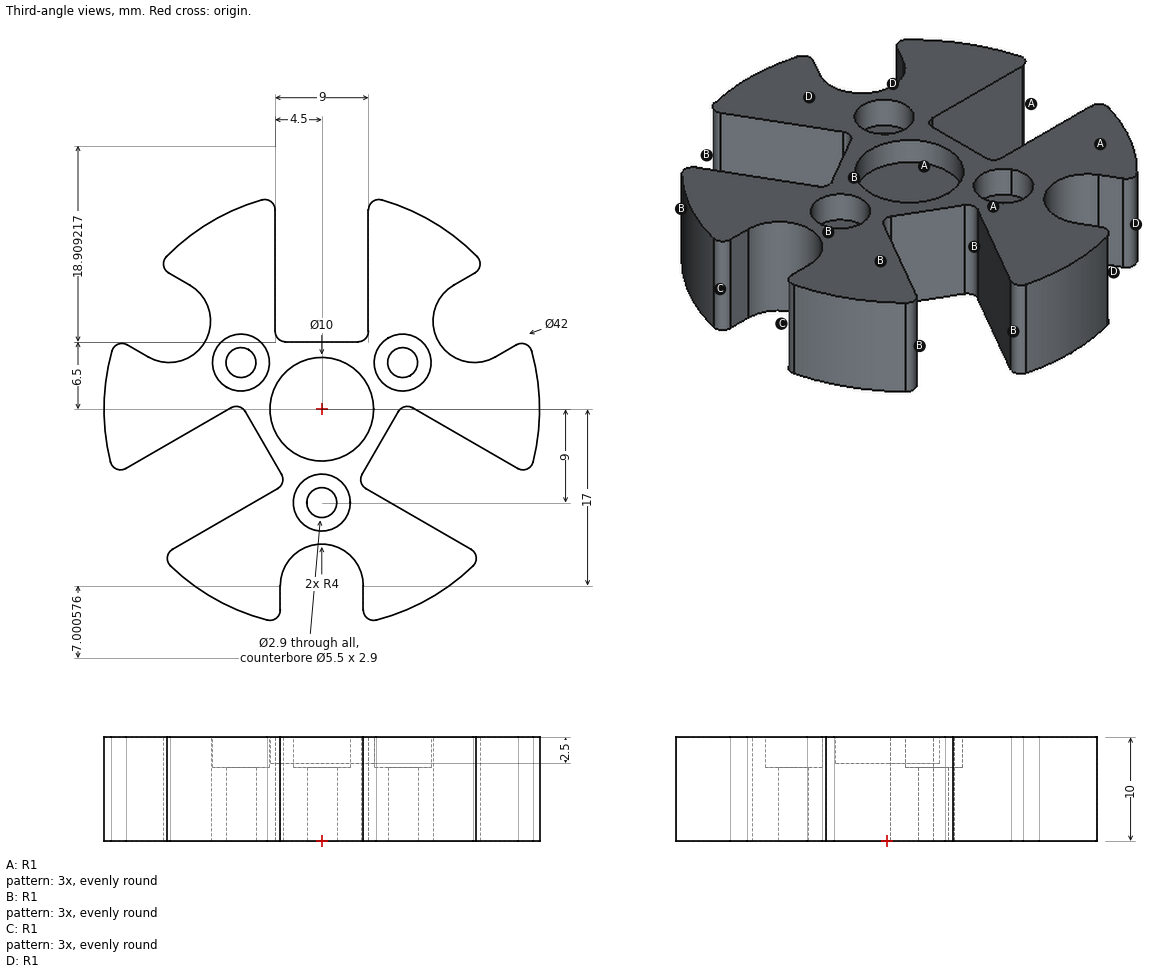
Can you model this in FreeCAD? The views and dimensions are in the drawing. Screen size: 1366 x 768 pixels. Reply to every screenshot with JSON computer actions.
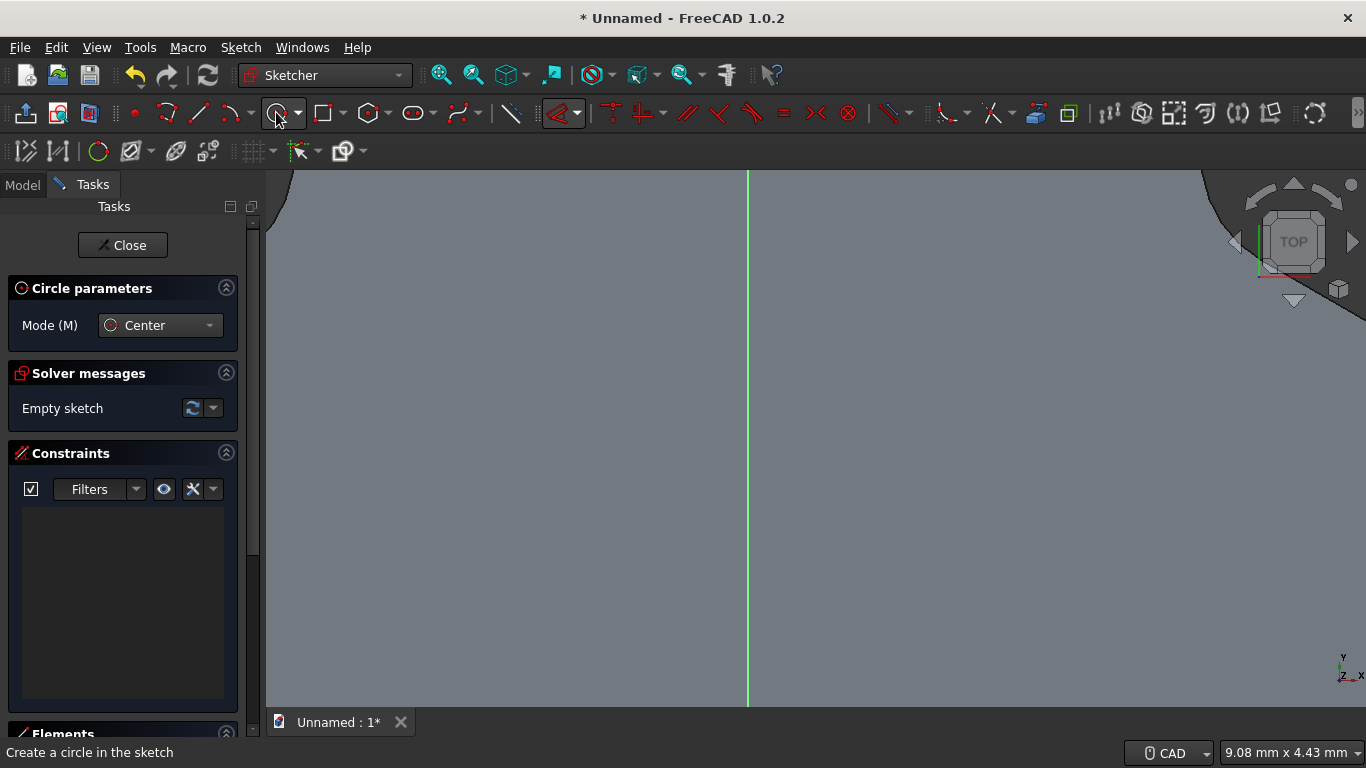
{"action": "left_click", "coordinate": [748, 424]}
{"action": "left_click", "coordinate": [872, 300]}
{"action": "key", "text": "Escape"}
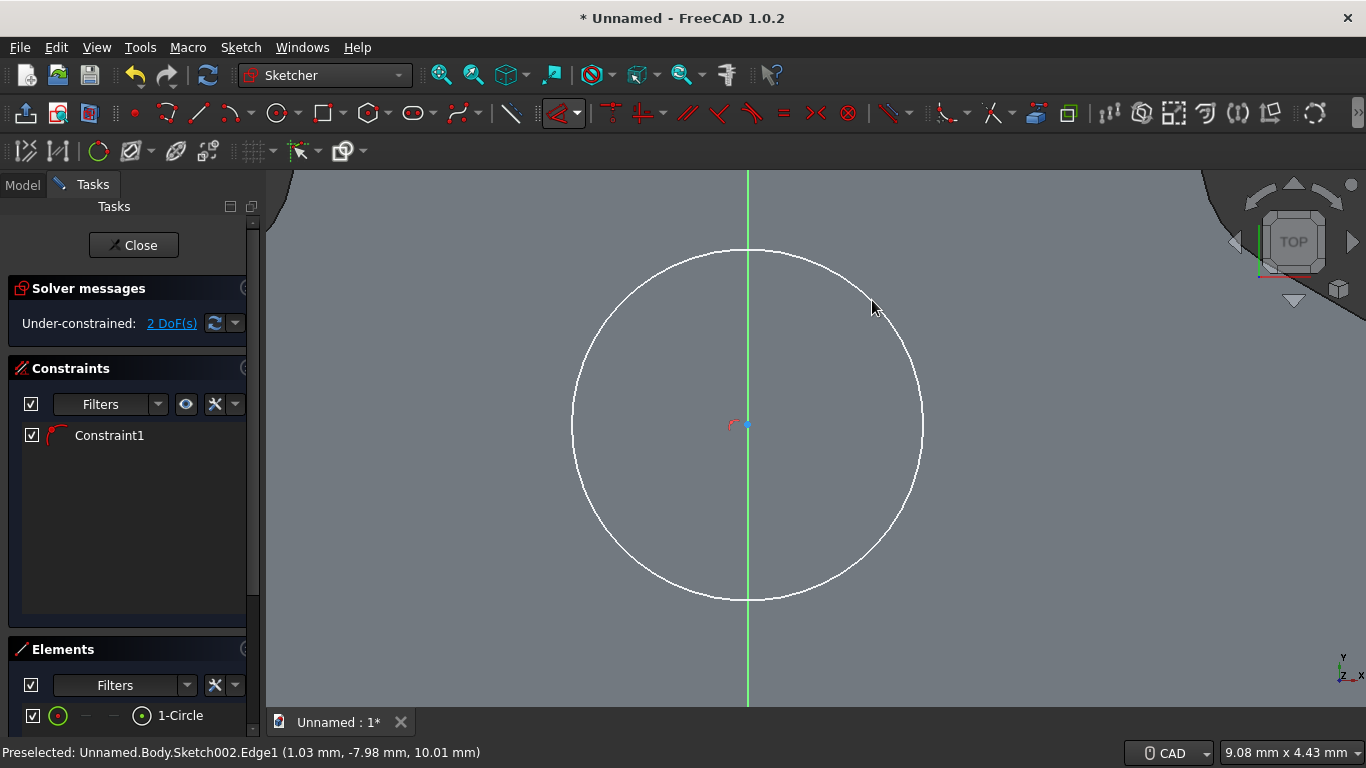
{"action": "left_click", "coordinate": [871, 300]}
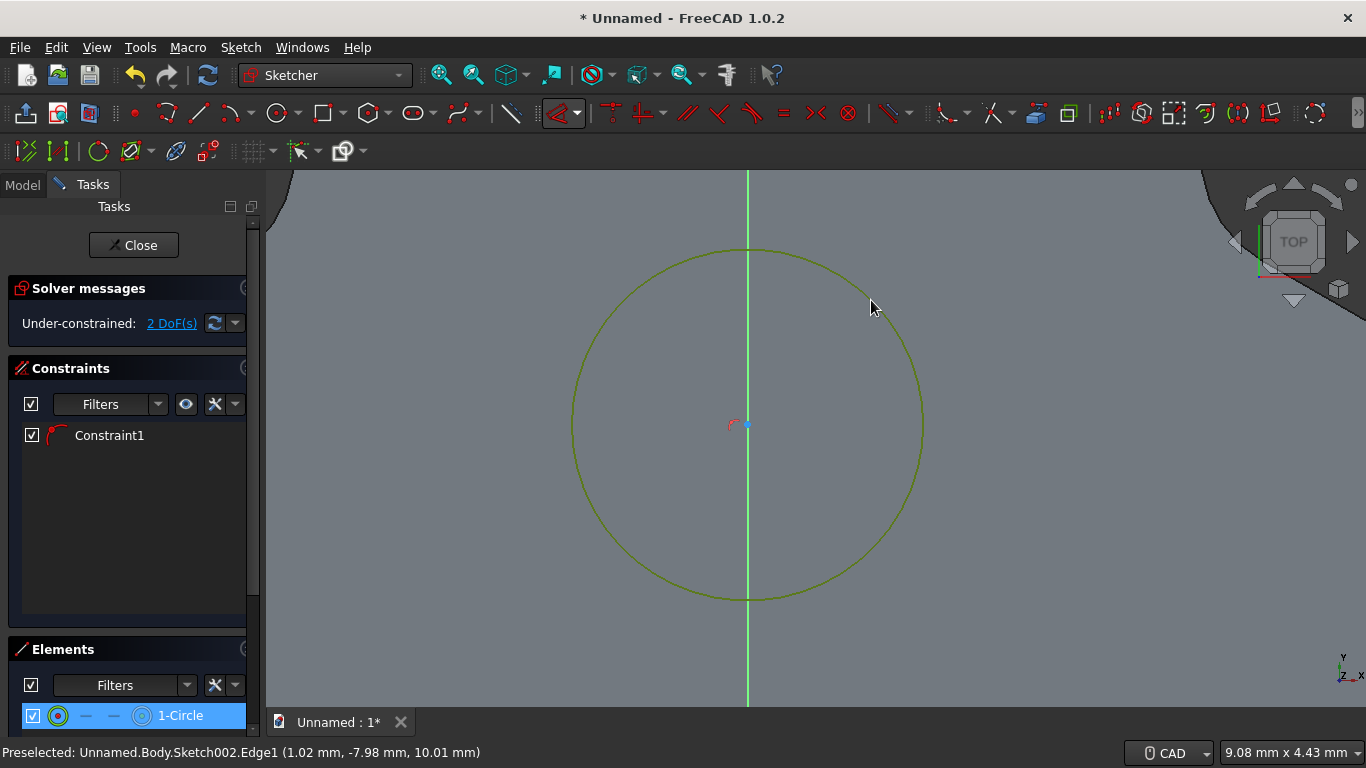
{"action": "left_click", "coordinate": [580, 114]}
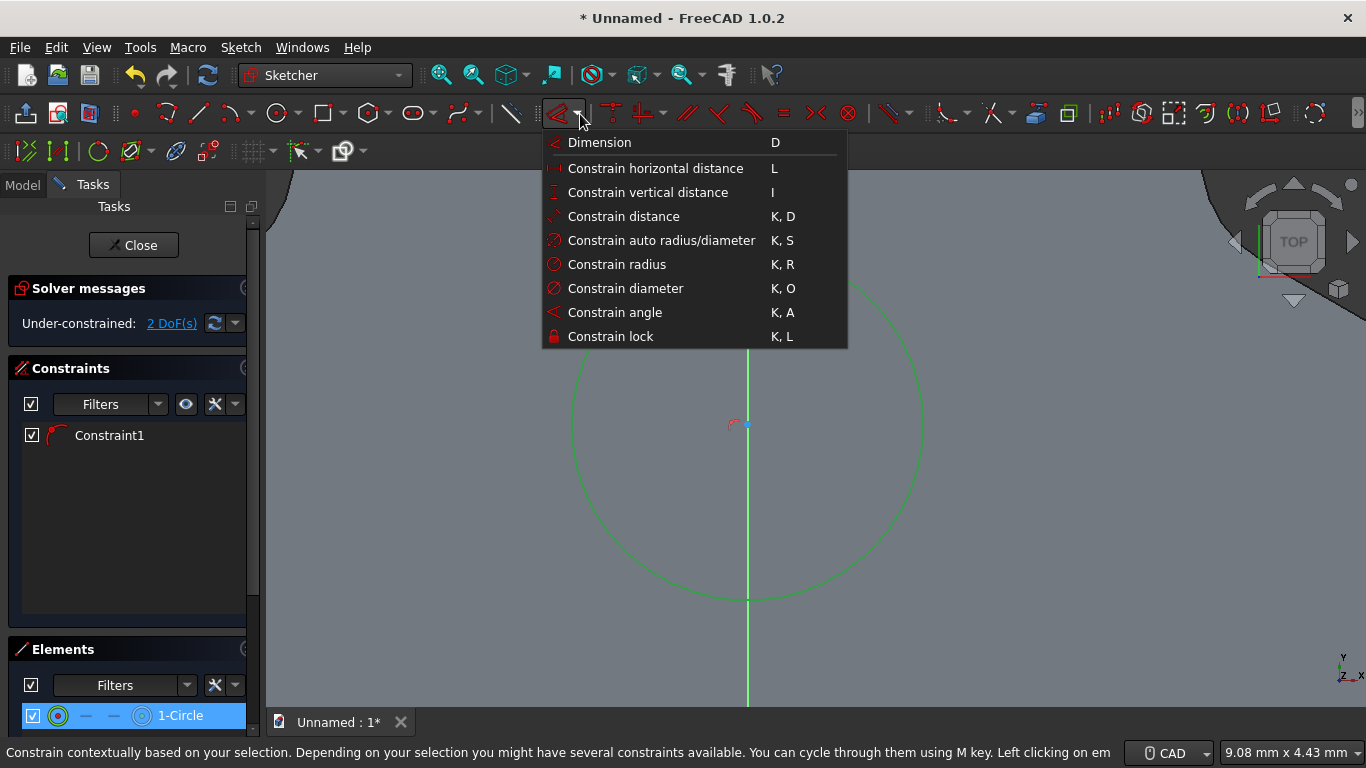
{"action": "left_click", "coordinate": [695, 288]}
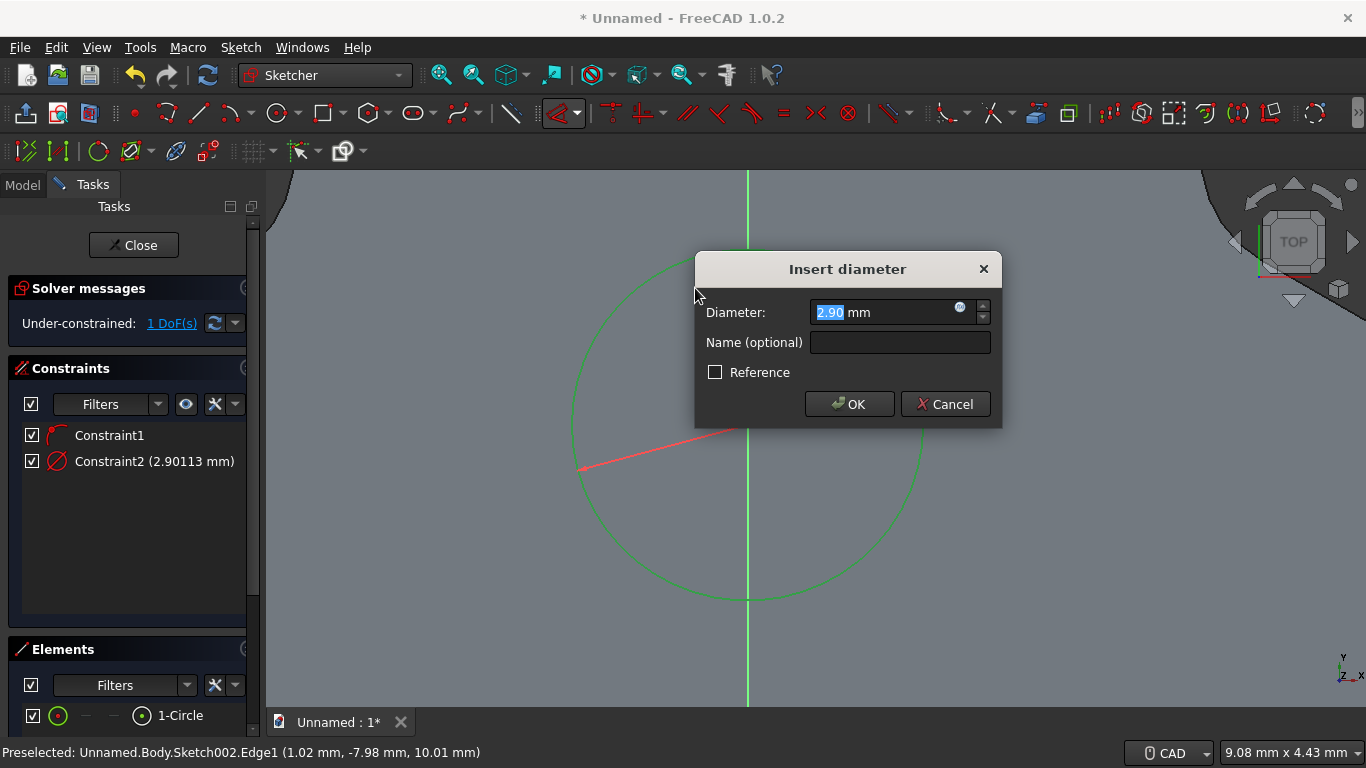
{"action": "type", "text": "2.9"}
{"action": "key", "text": "Return"}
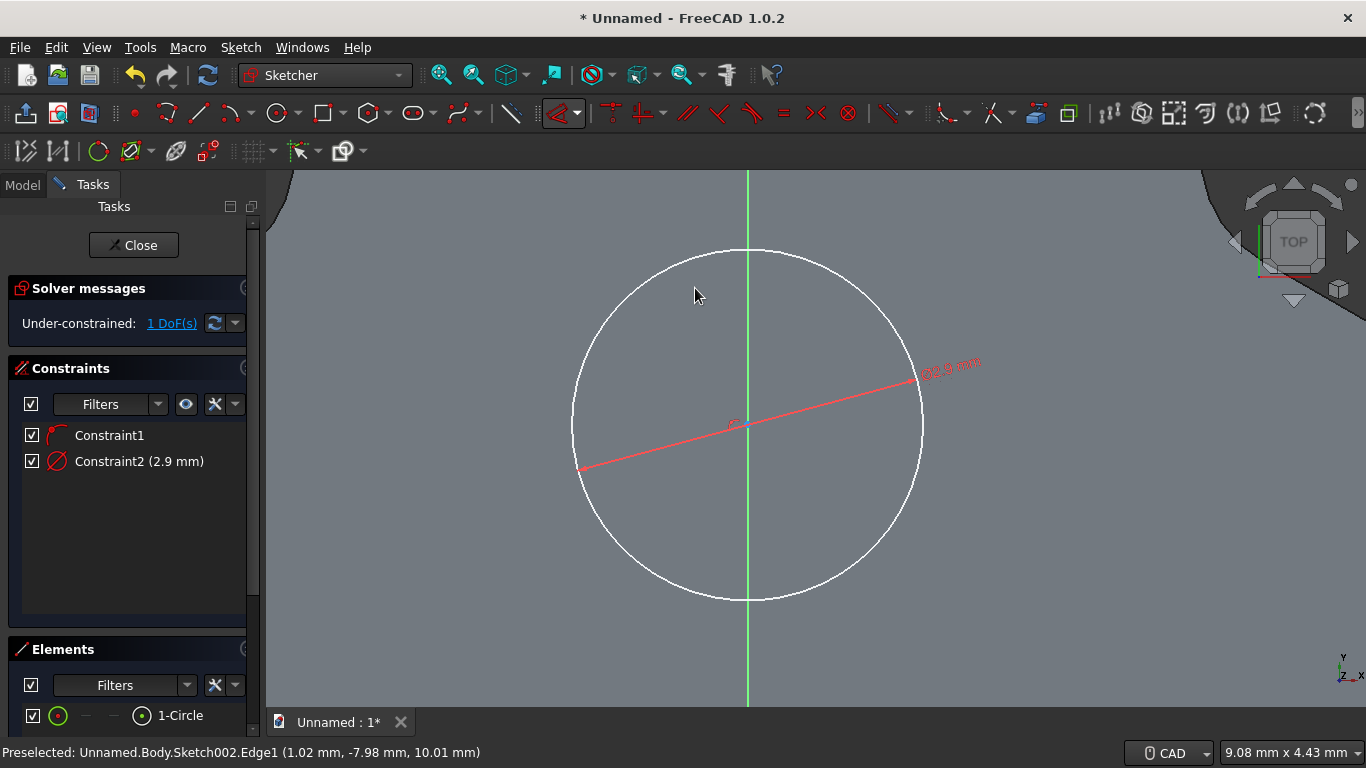
{"action": "left_click", "coordinate": [748, 425]}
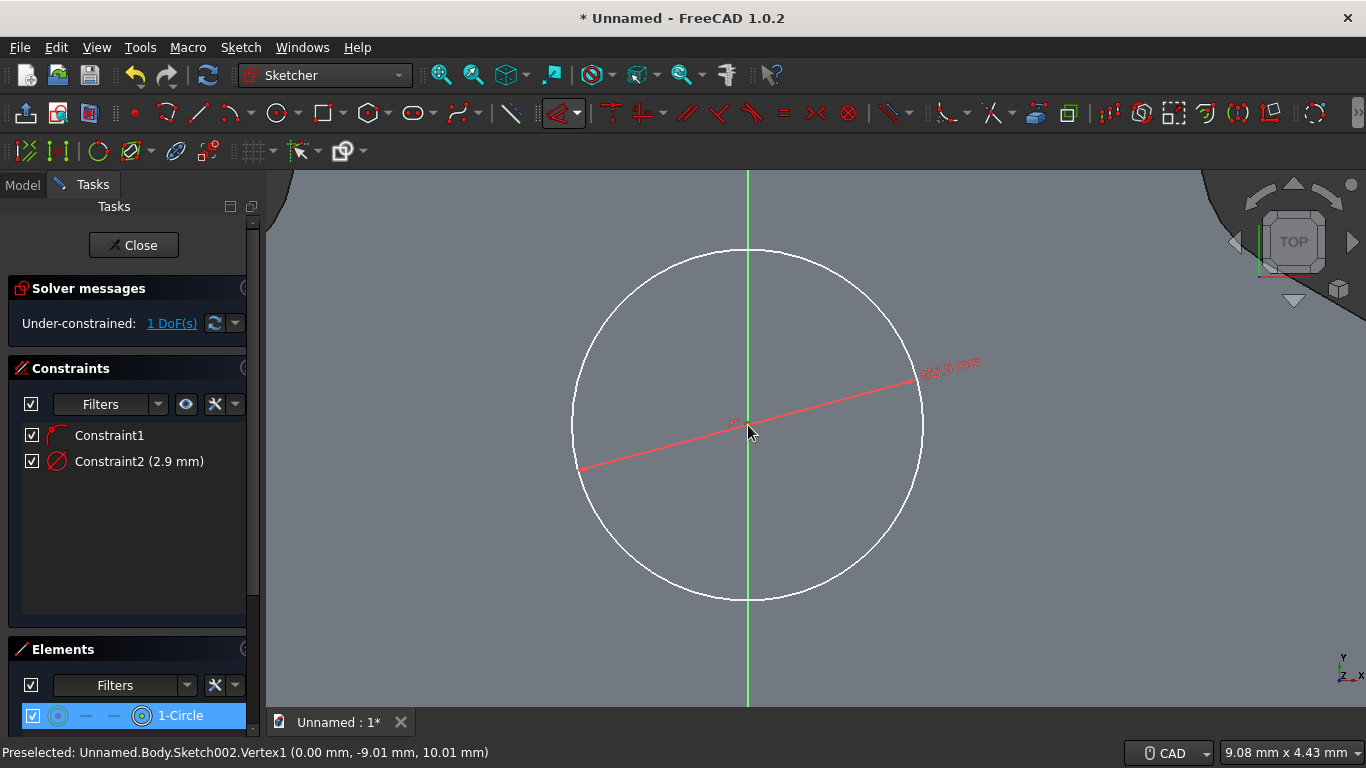
{"action": "left_click", "coordinate": [580, 114]}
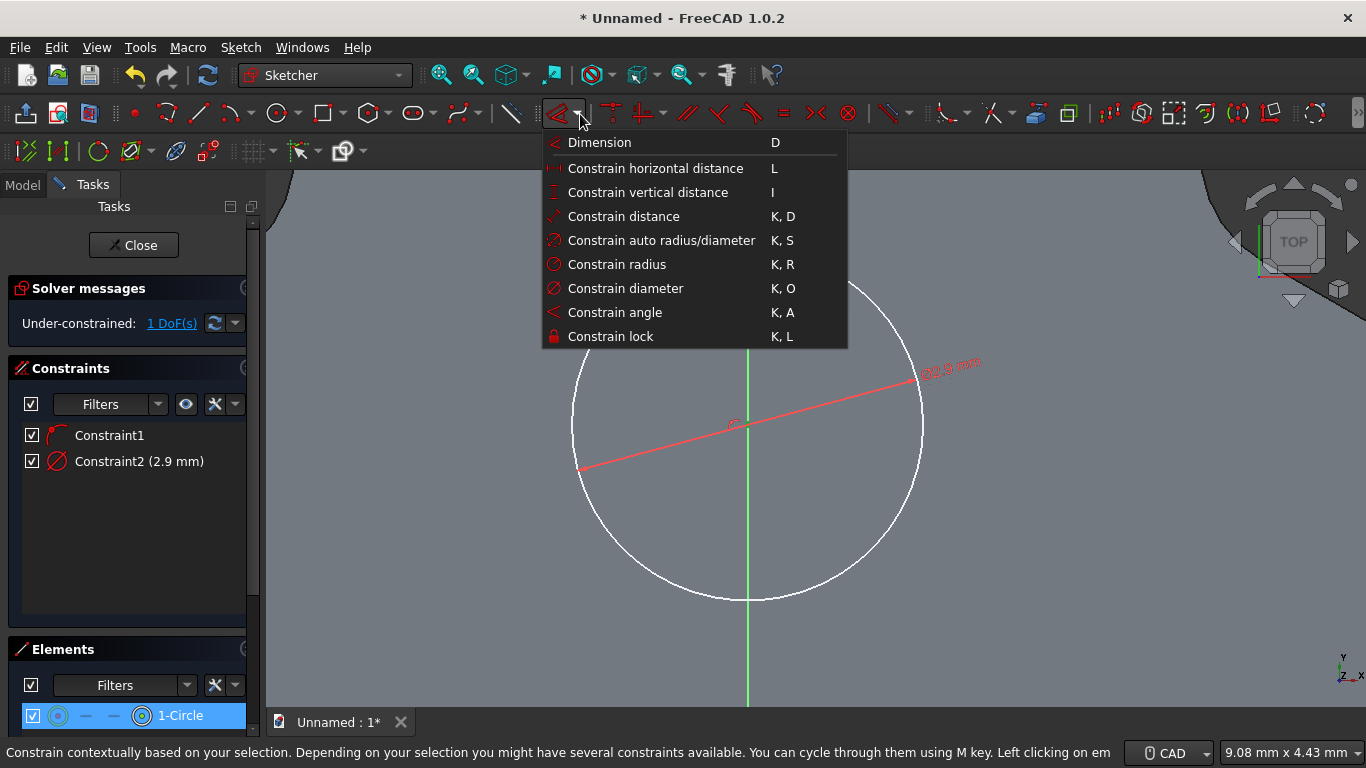
{"action": "left_click", "coordinate": [695, 192]}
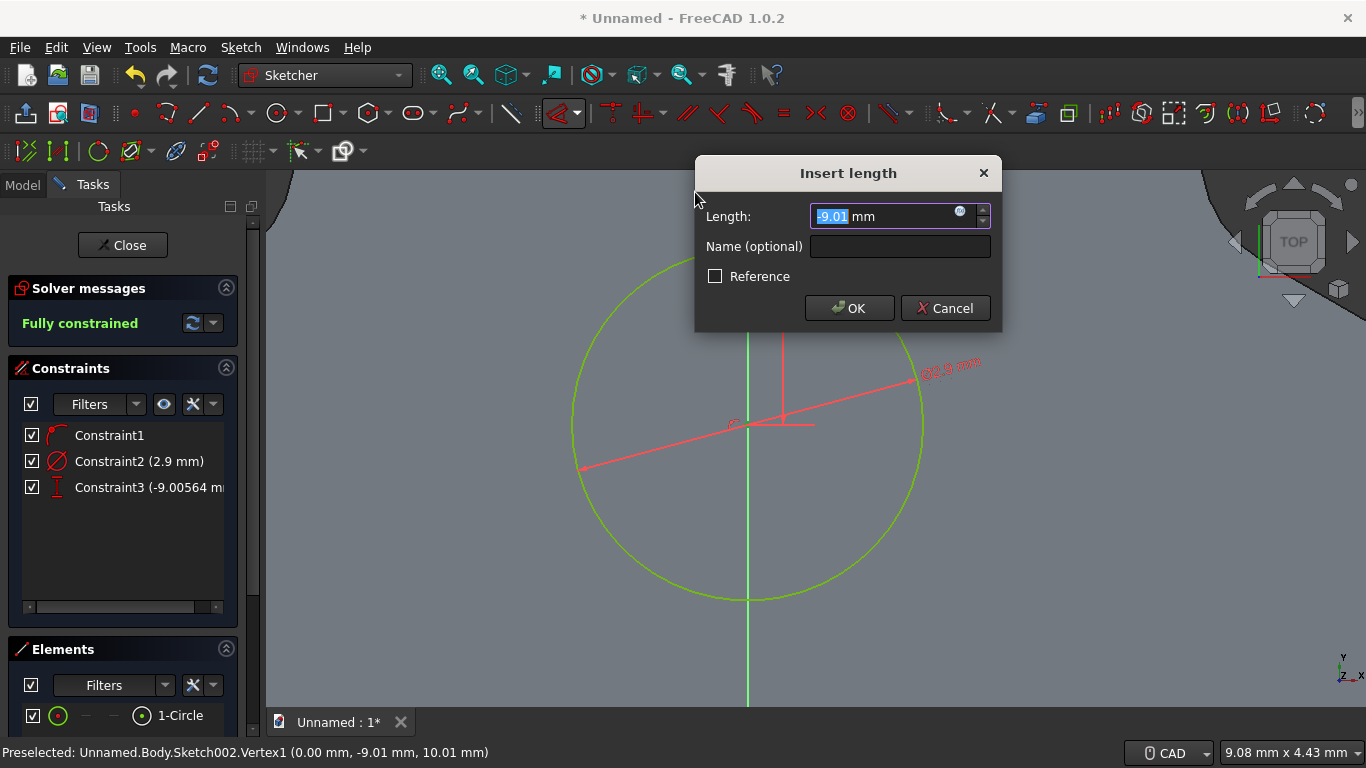
{"action": "type", "text": "-9"}
{"action": "key", "text": "Return"}